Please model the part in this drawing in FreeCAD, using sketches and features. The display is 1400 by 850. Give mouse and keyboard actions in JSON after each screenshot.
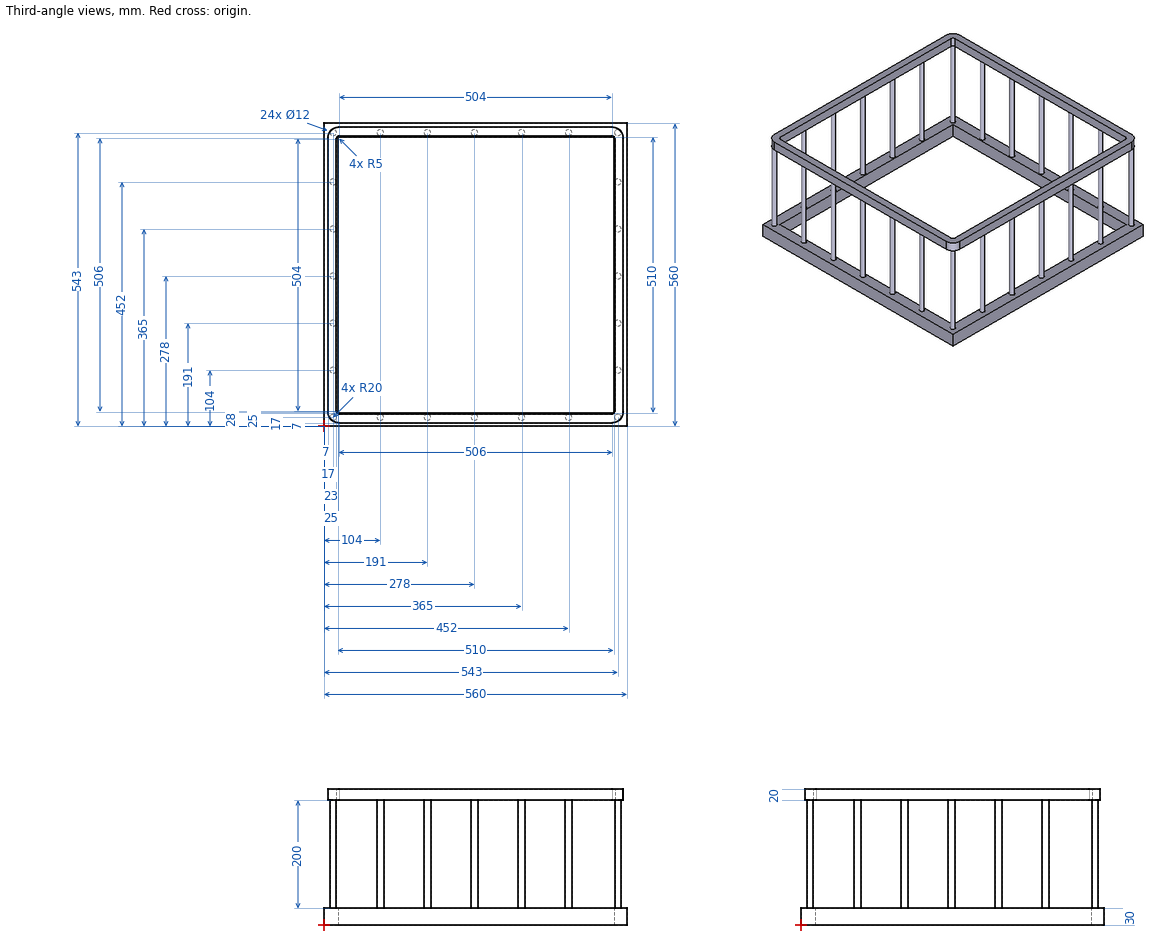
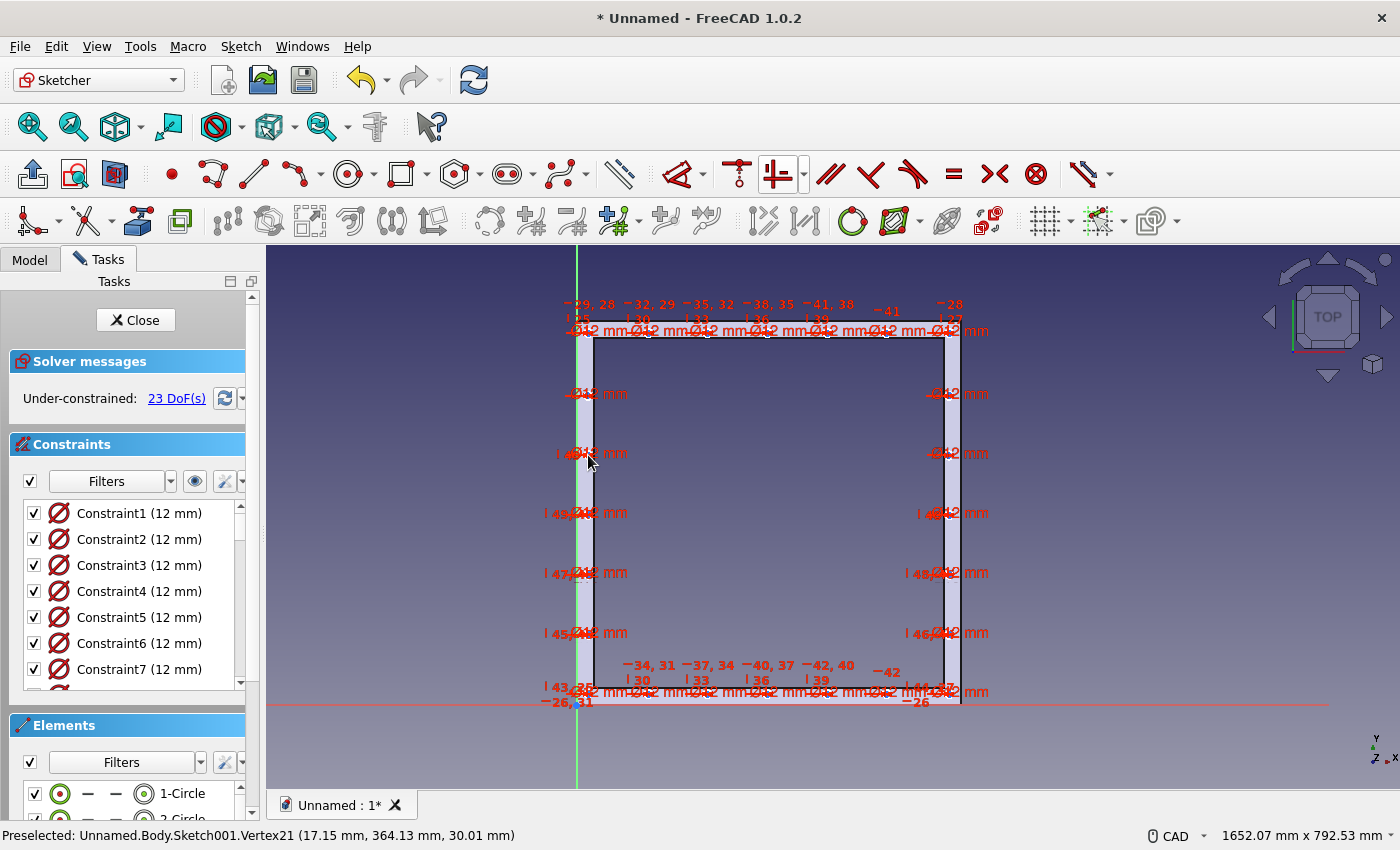
{"action": "left_click", "coordinate": [949, 515]}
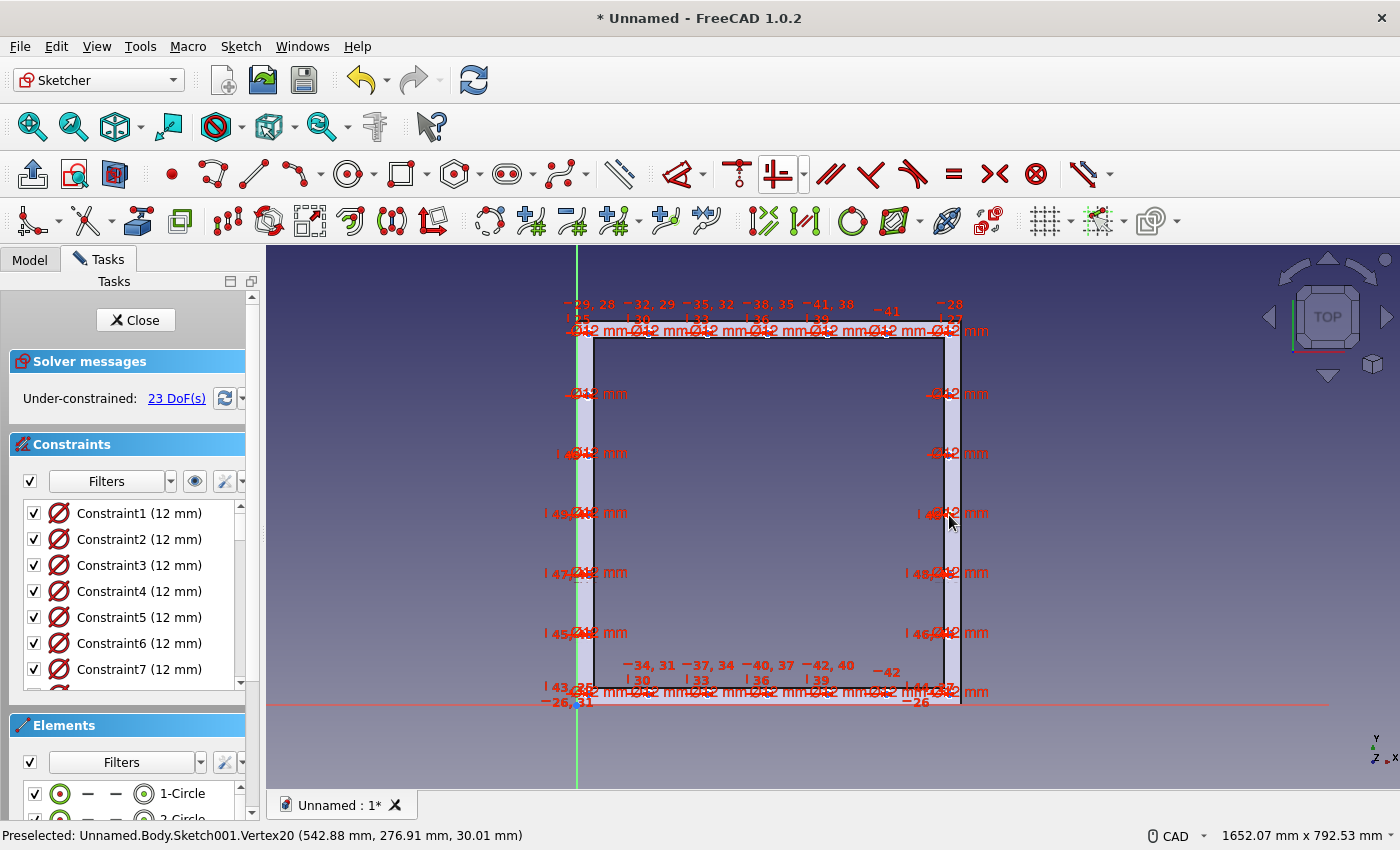
{"action": "left_click", "coordinate": [949, 455]}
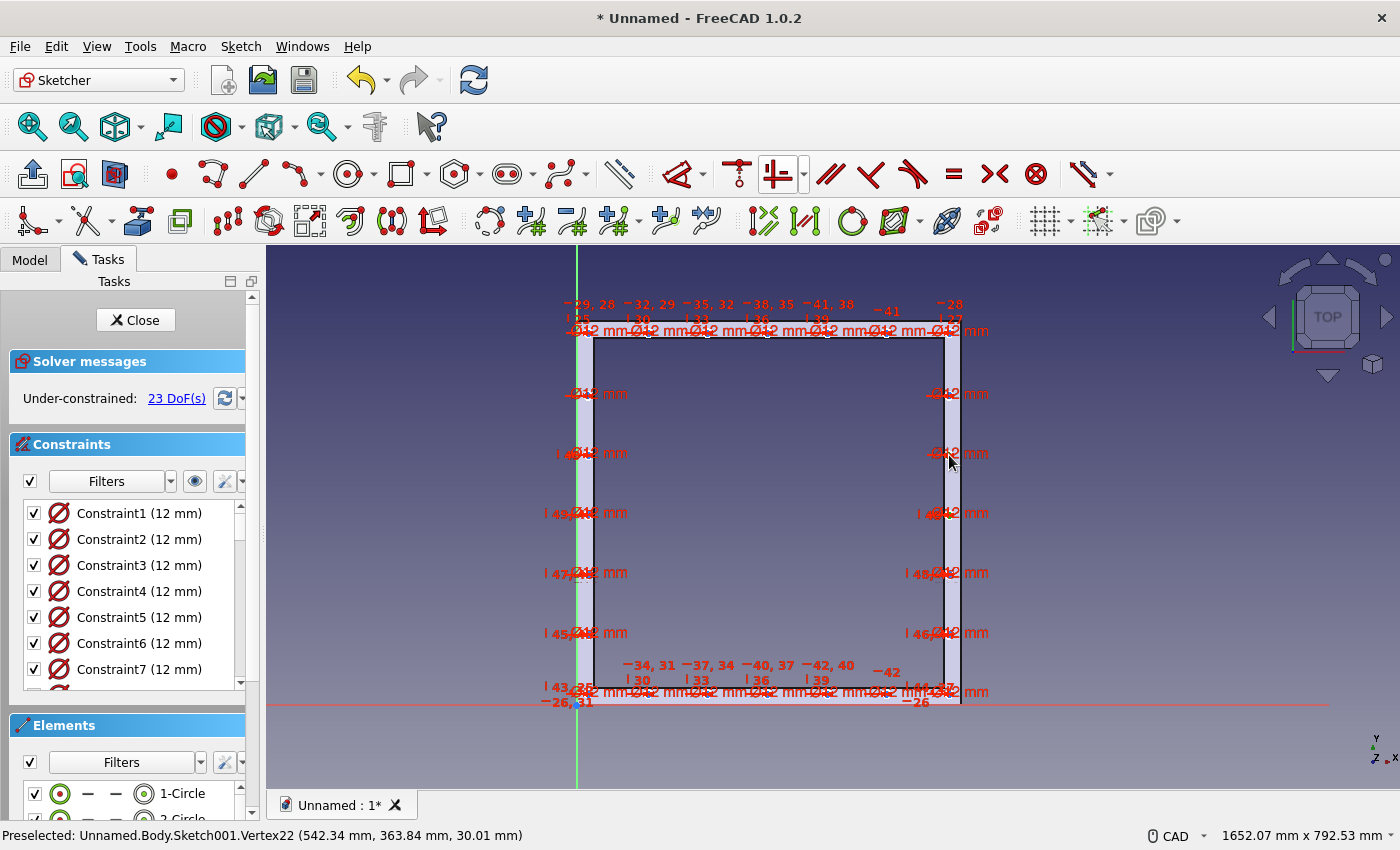
{"action": "key", "text": "v"}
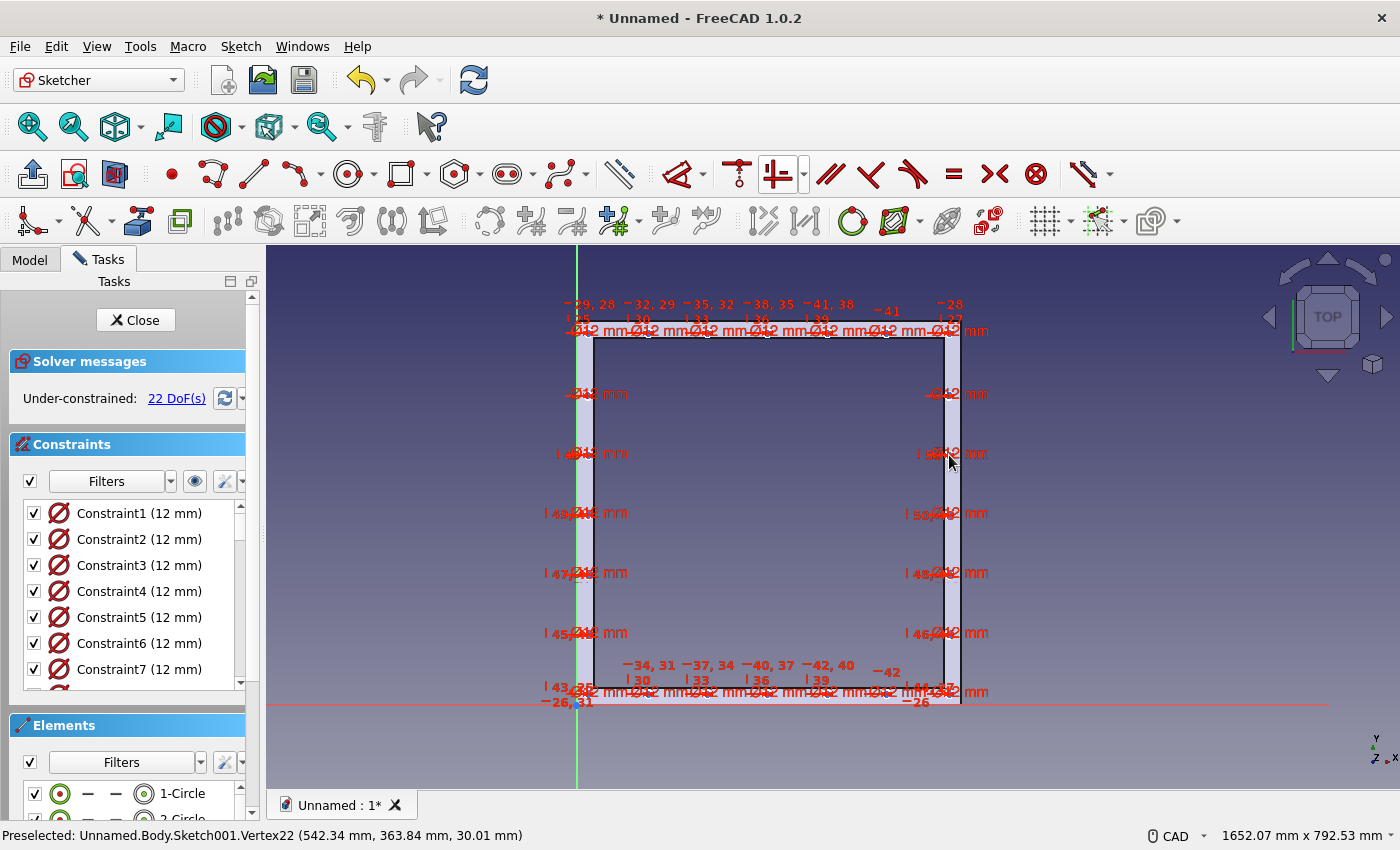
{"action": "left_click", "coordinate": [588, 455]}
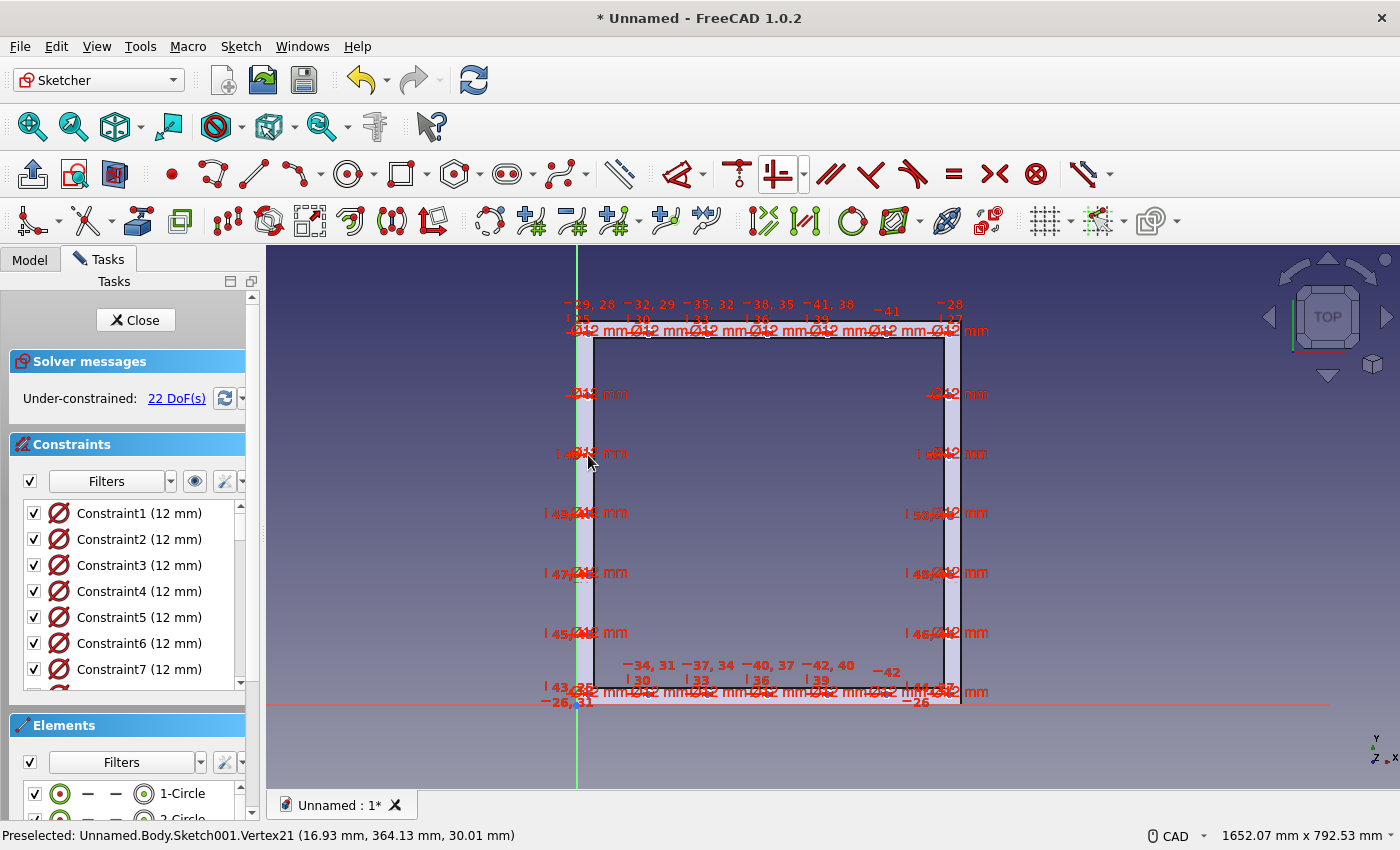
{"action": "left_click", "coordinate": [588, 396]}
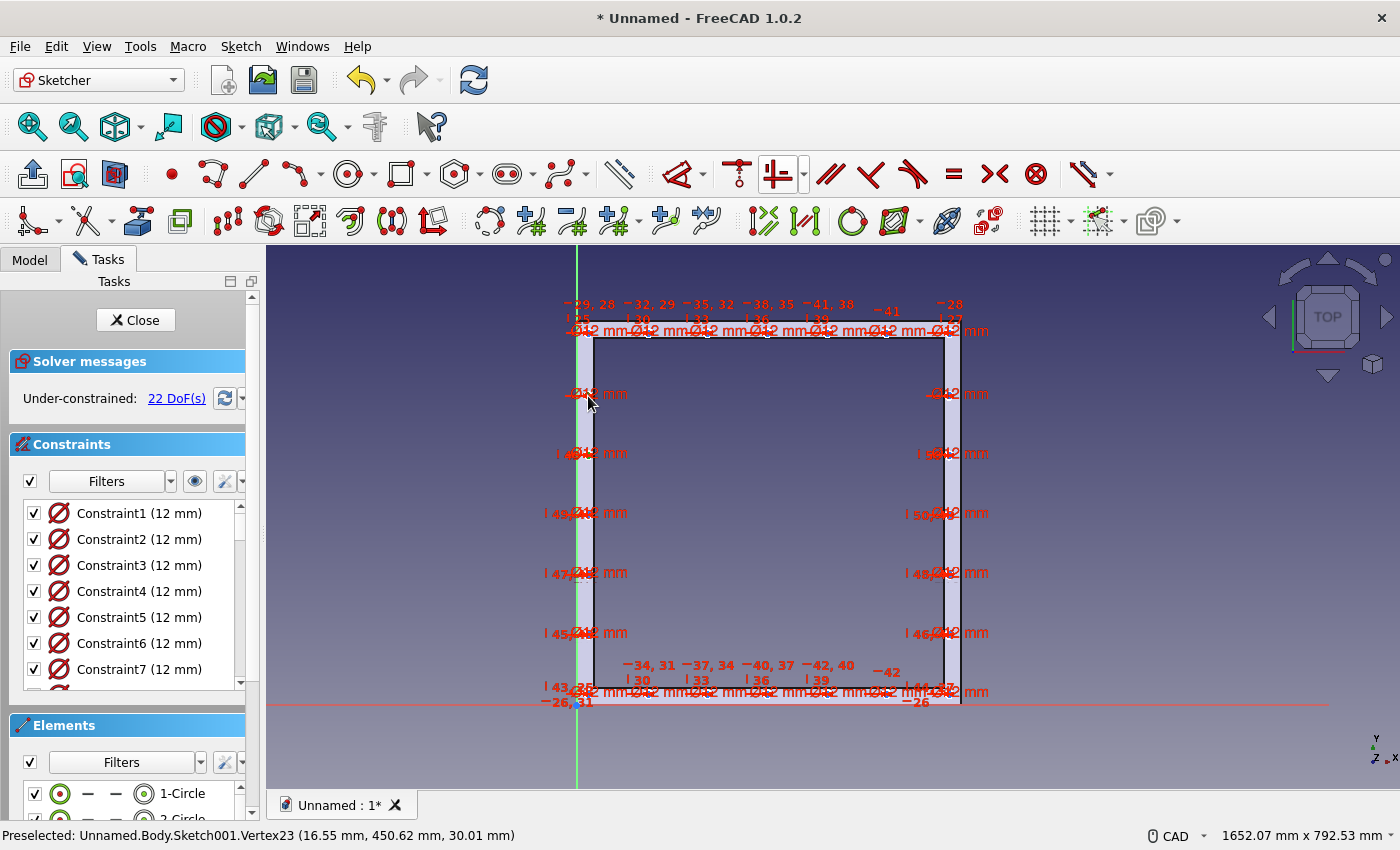
{"action": "key", "text": "v"}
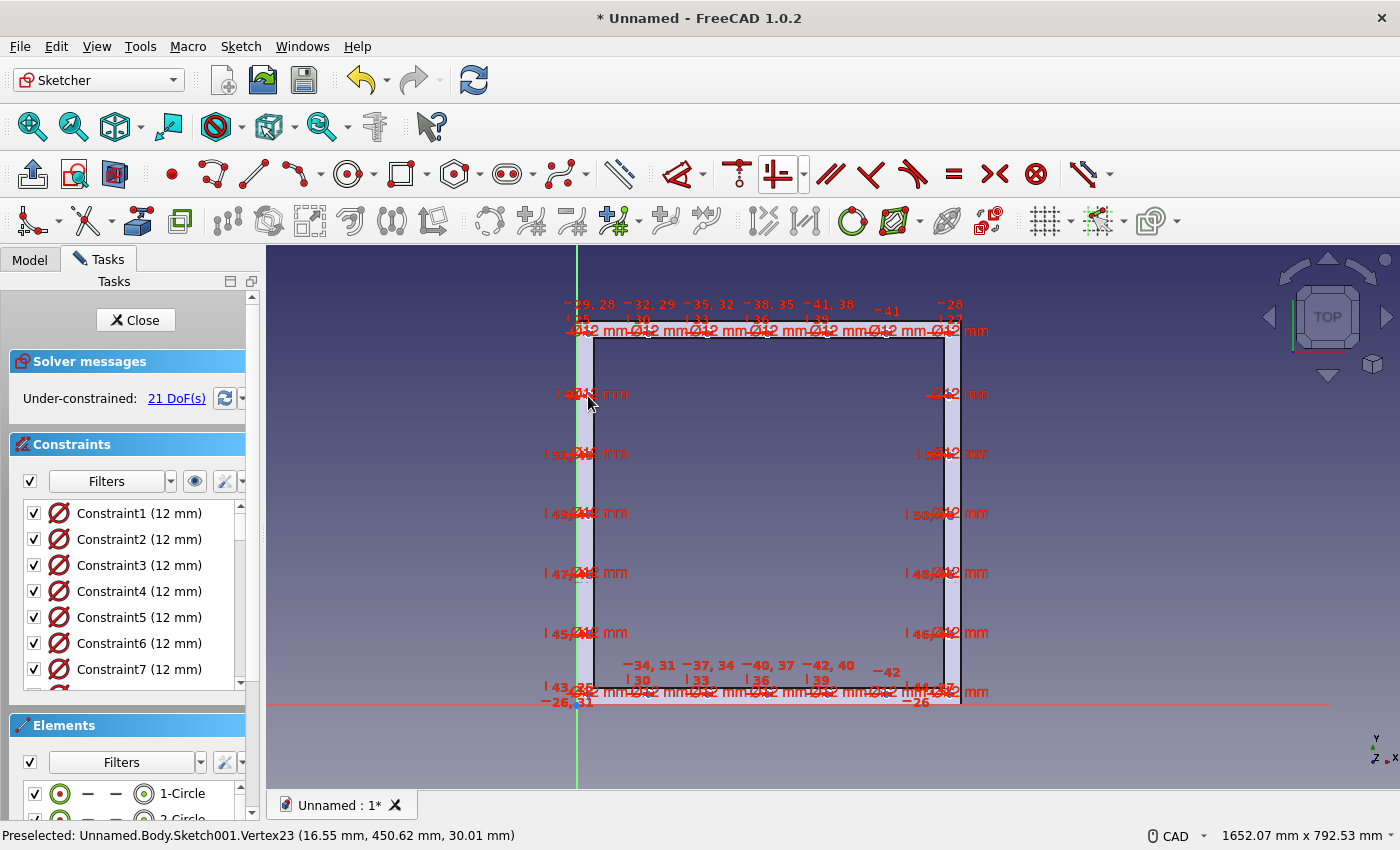
{"action": "left_click", "coordinate": [949, 455]}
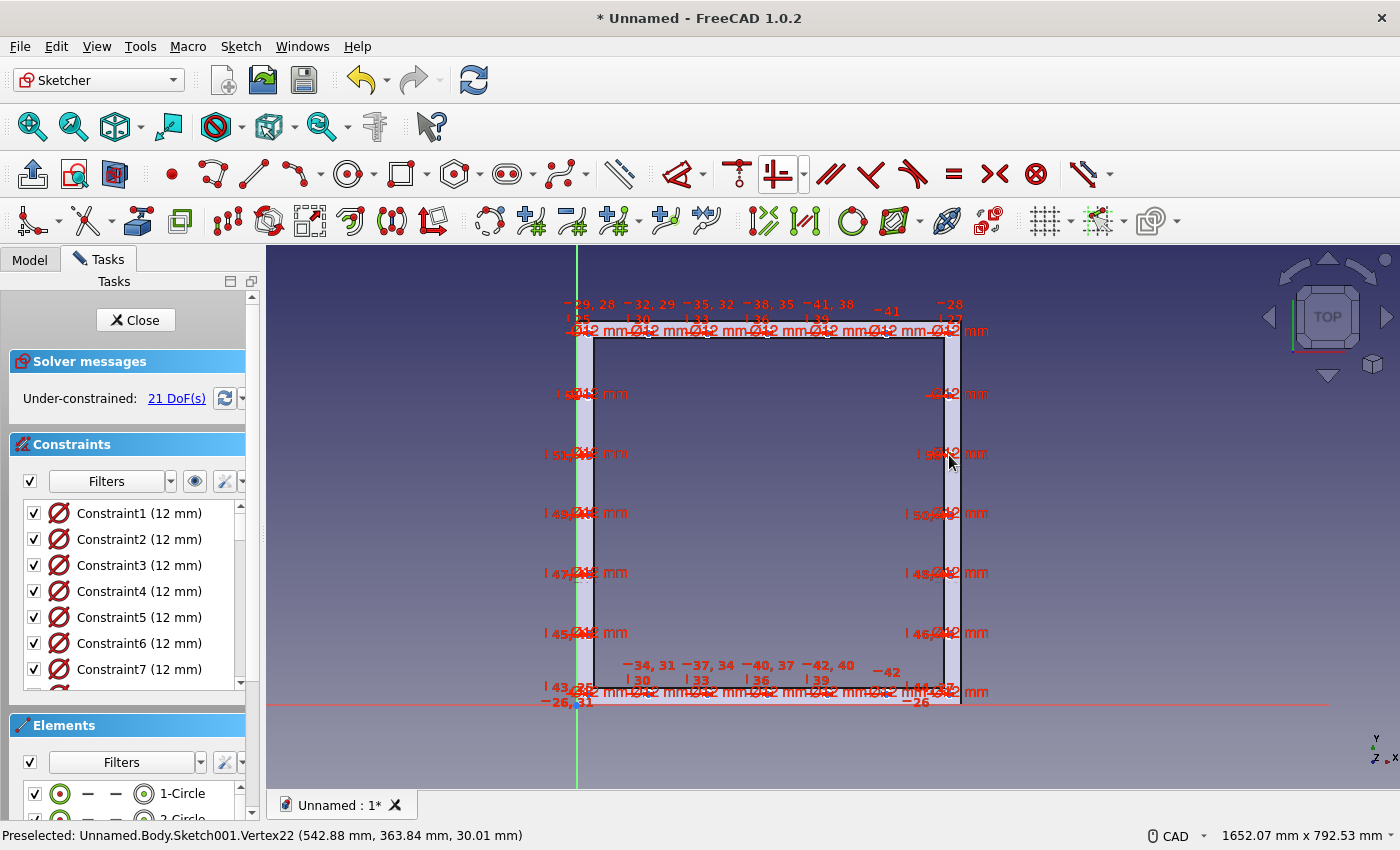
{"action": "left_click", "coordinate": [949, 396]}